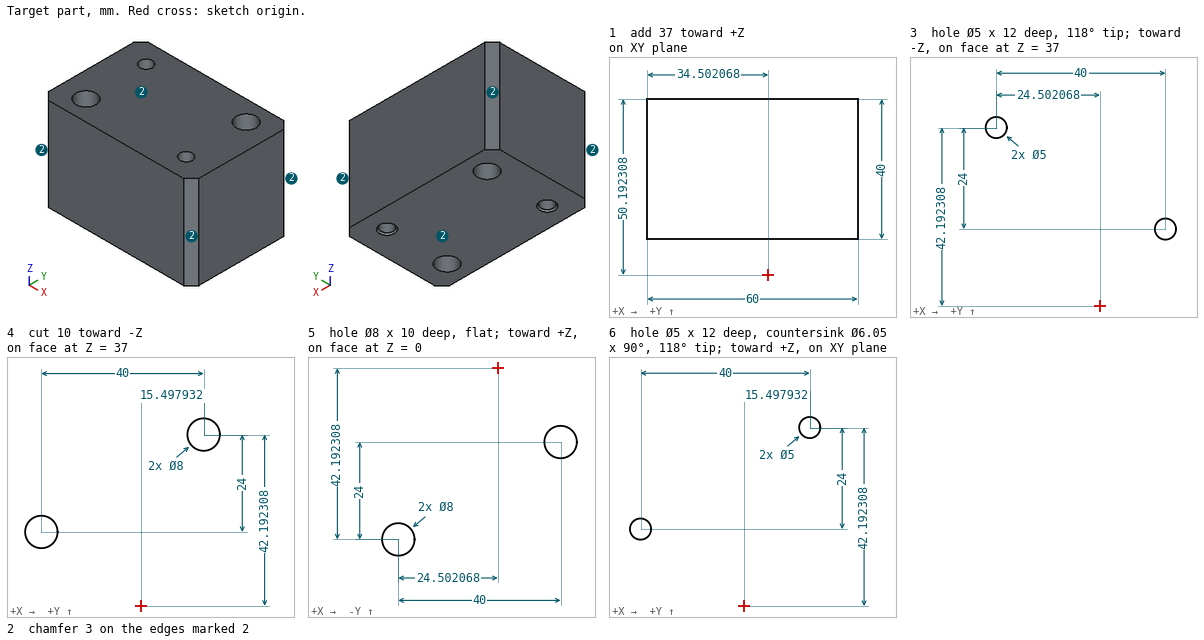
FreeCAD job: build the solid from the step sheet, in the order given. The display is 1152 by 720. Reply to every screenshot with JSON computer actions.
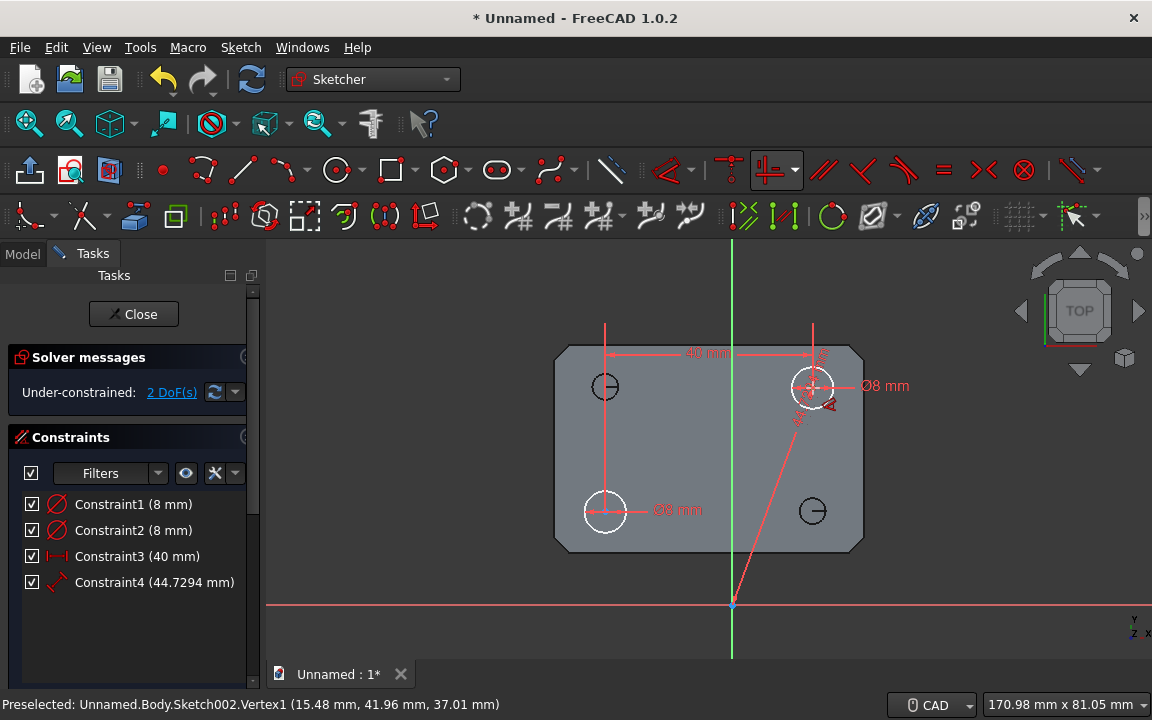
{"action": "left_click", "coordinate": [605, 512]}
{"action": "left_click", "coordinate": [571, 450]}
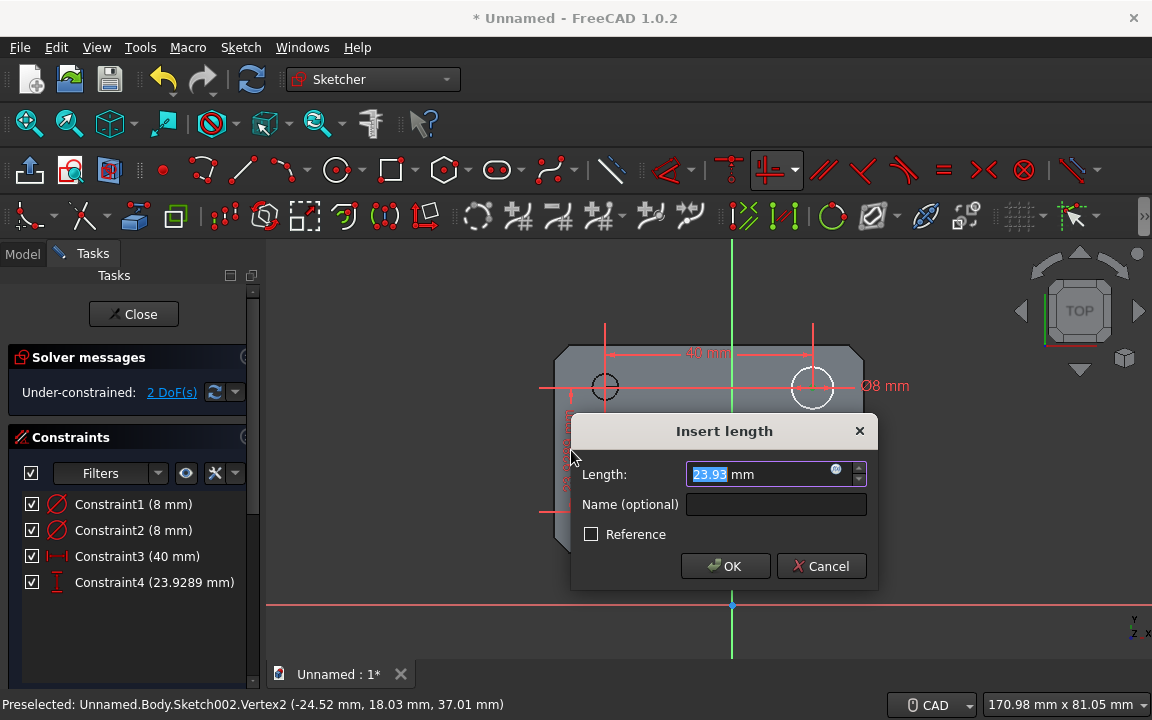
{"action": "type", "text": "24"}
{"action": "key", "text": "Return"}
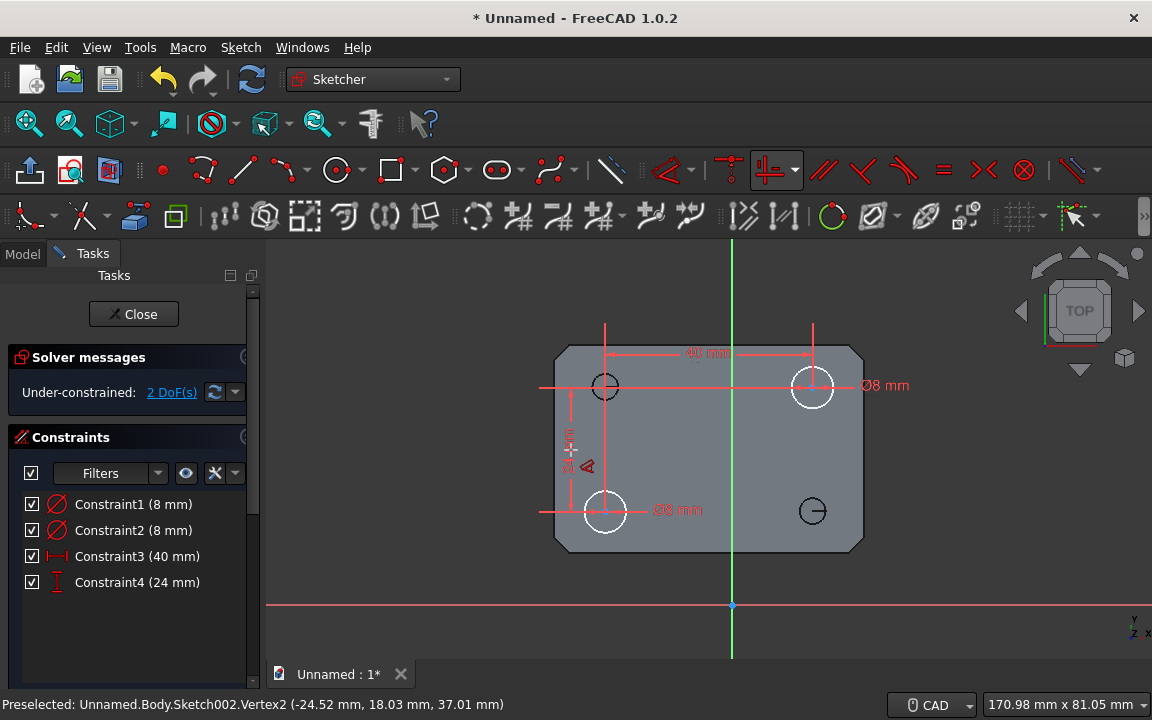
{"action": "left_click", "coordinate": [813, 388]}
{"action": "left_click", "coordinate": [791, 354]}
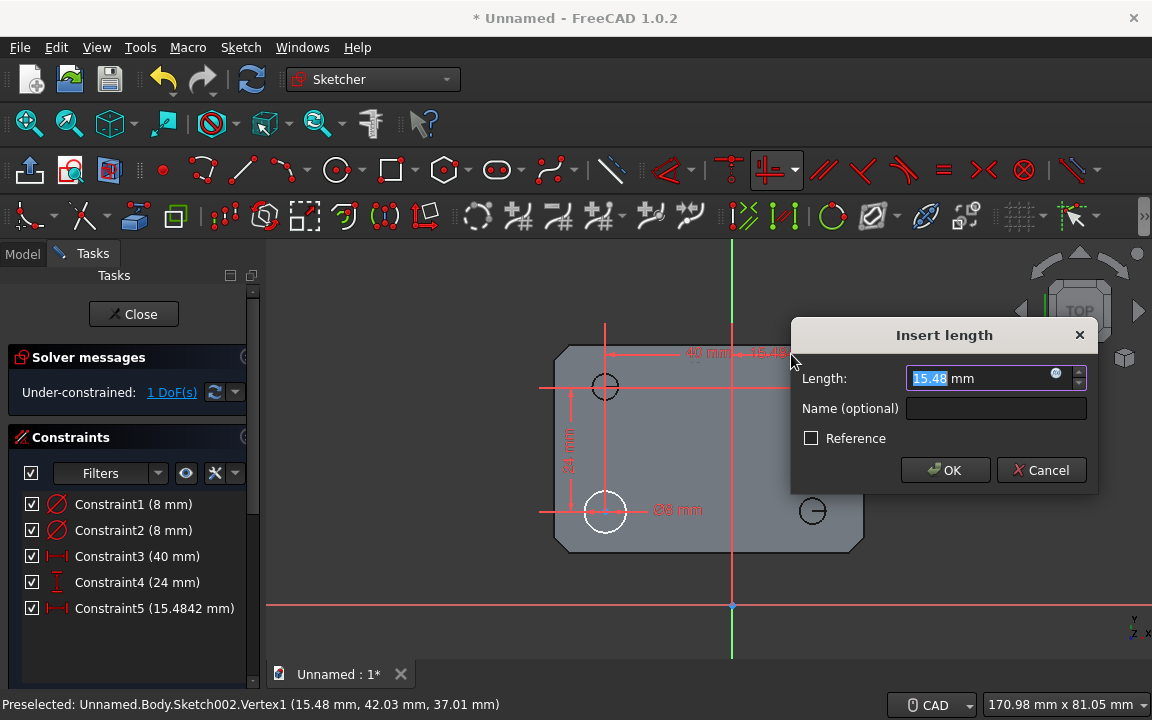
{"action": "type", "text": "15.497932"}
{"action": "key", "text": "Return"}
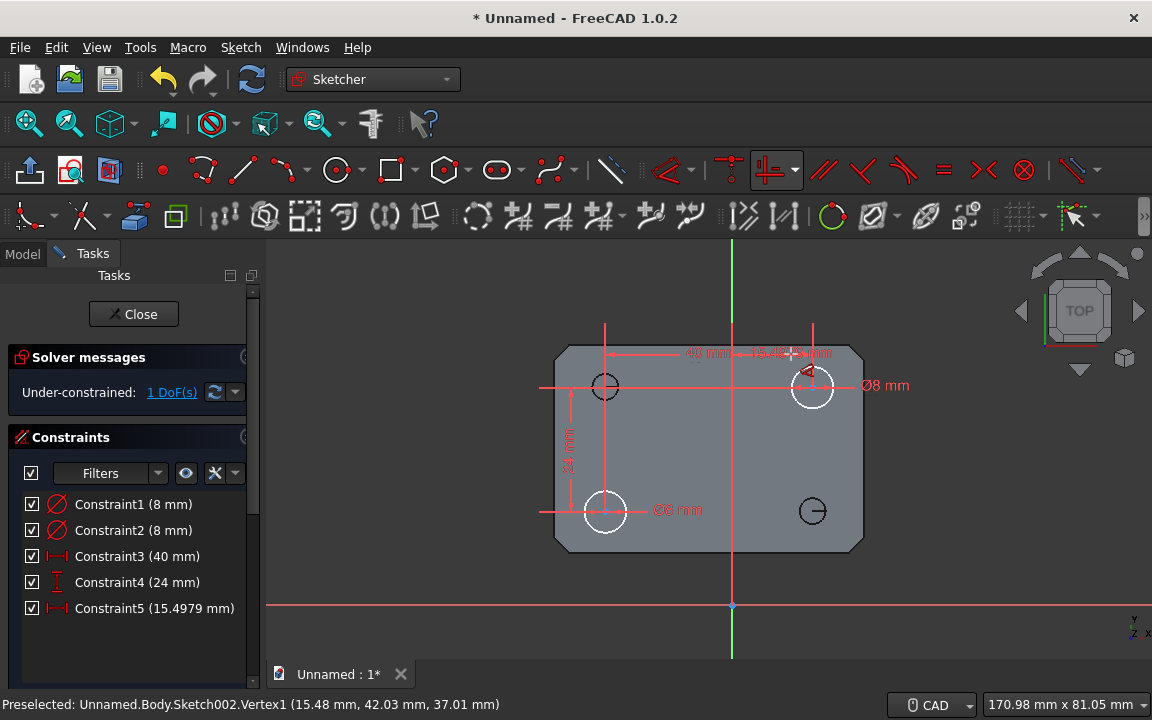
{"action": "left_click", "coordinate": [813, 388]}
{"action": "left_click", "coordinate": [847, 497]}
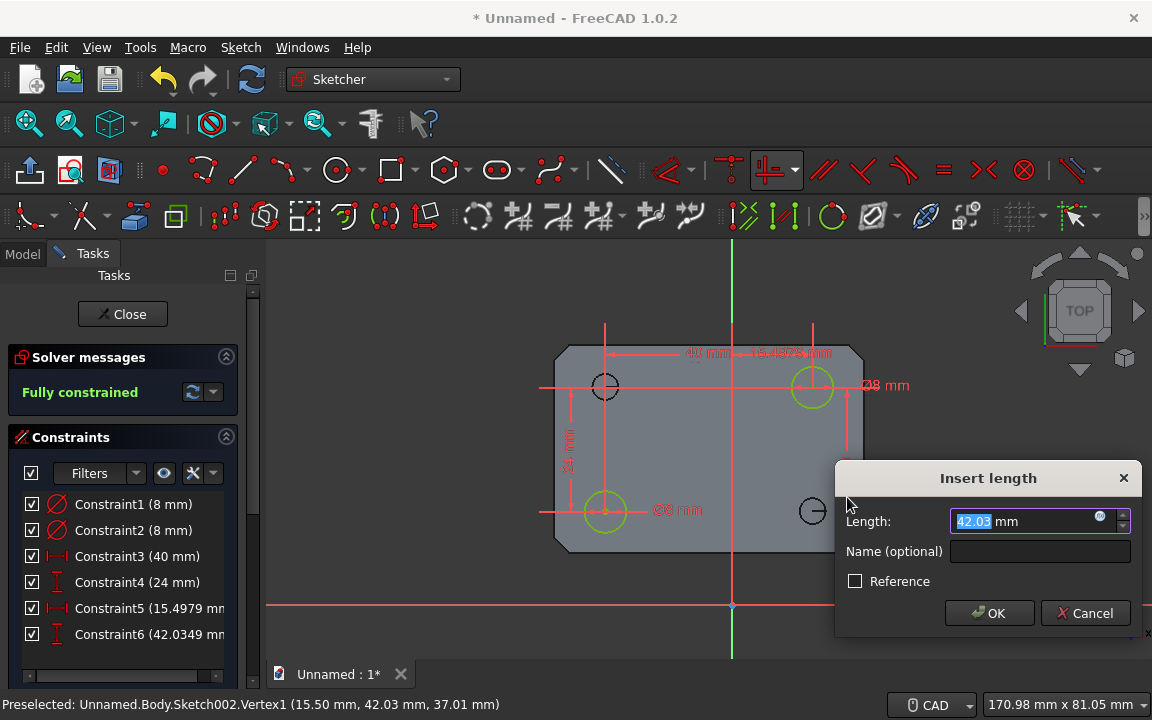
{"action": "type", "text": "42.192308"}
{"action": "key", "text": "Return"}
{"action": "key", "text": "Escape"}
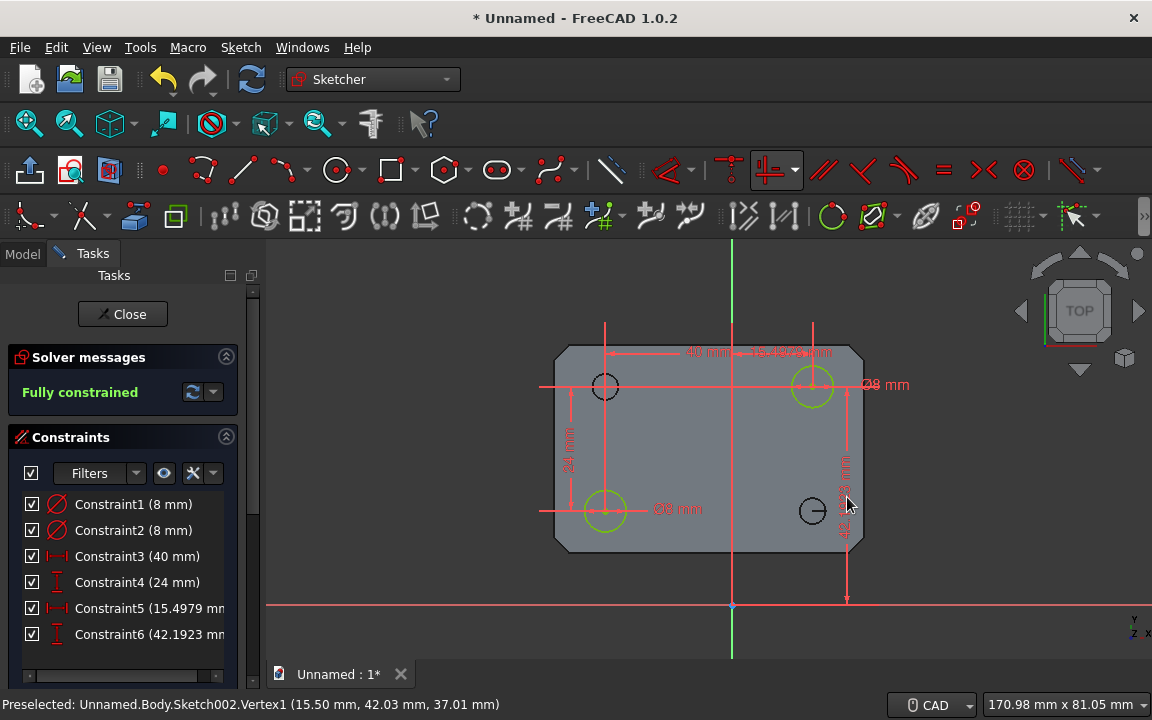
{"action": "left_click", "coordinate": [123, 314]}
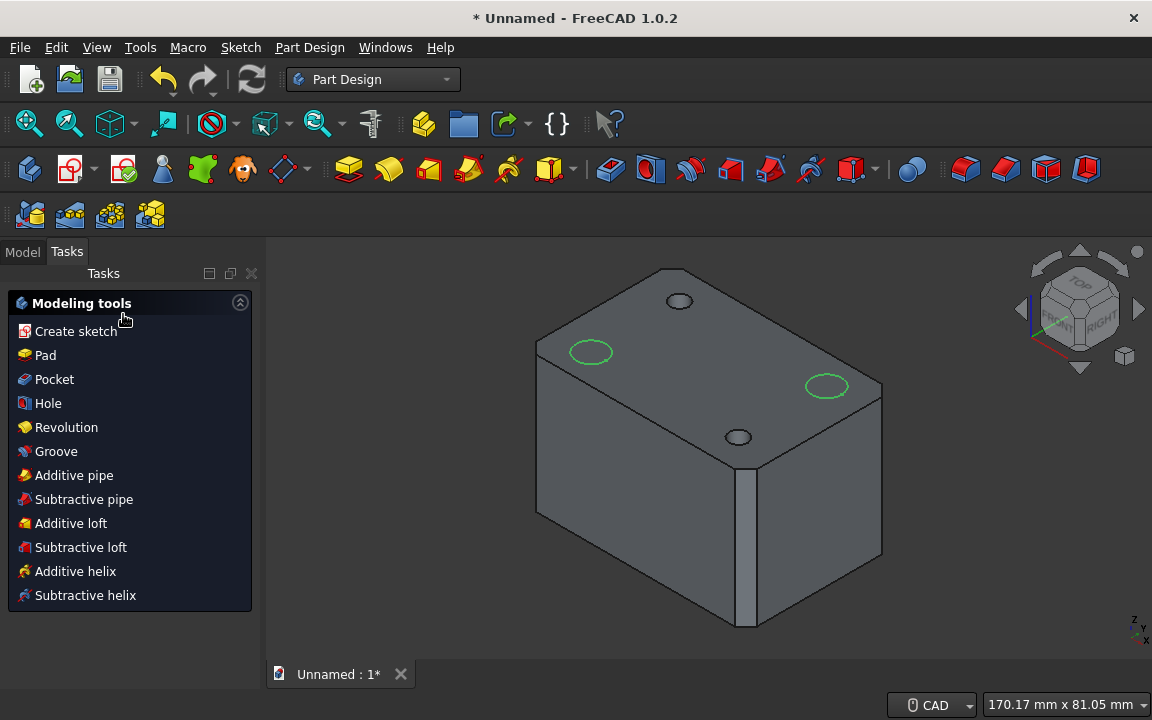
{"action": "left_click", "coordinate": [612, 170]}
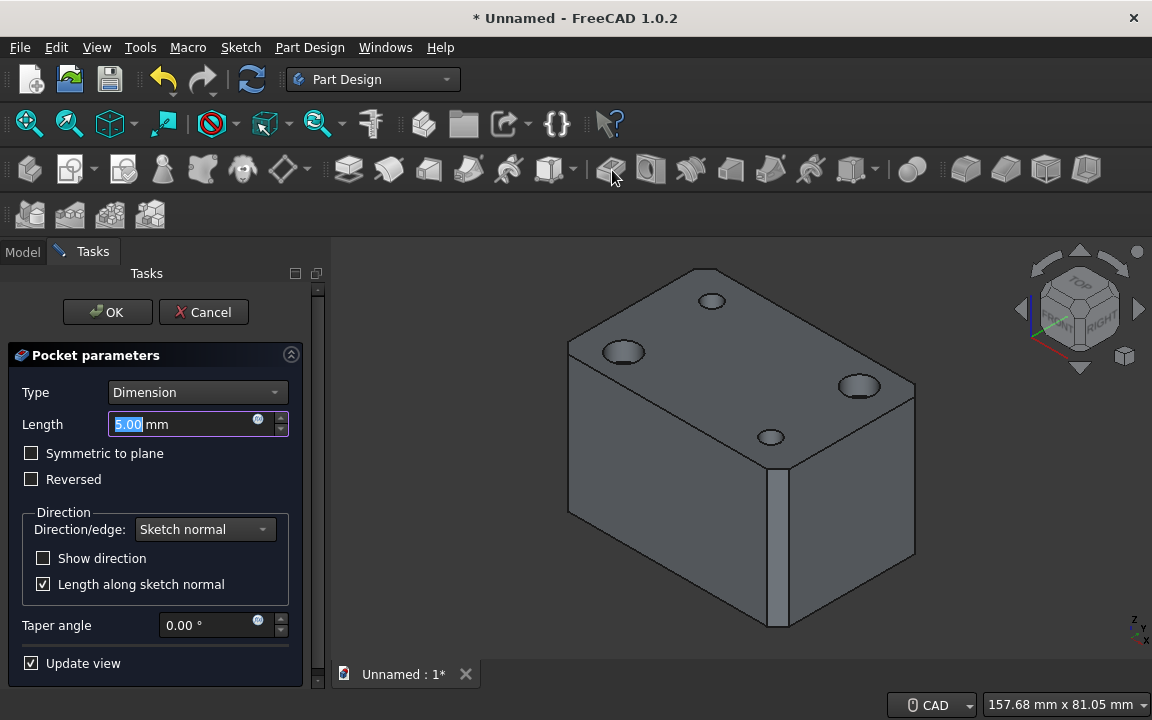
{"action": "type", "text": "10"}
{"action": "key", "text": "Tab"}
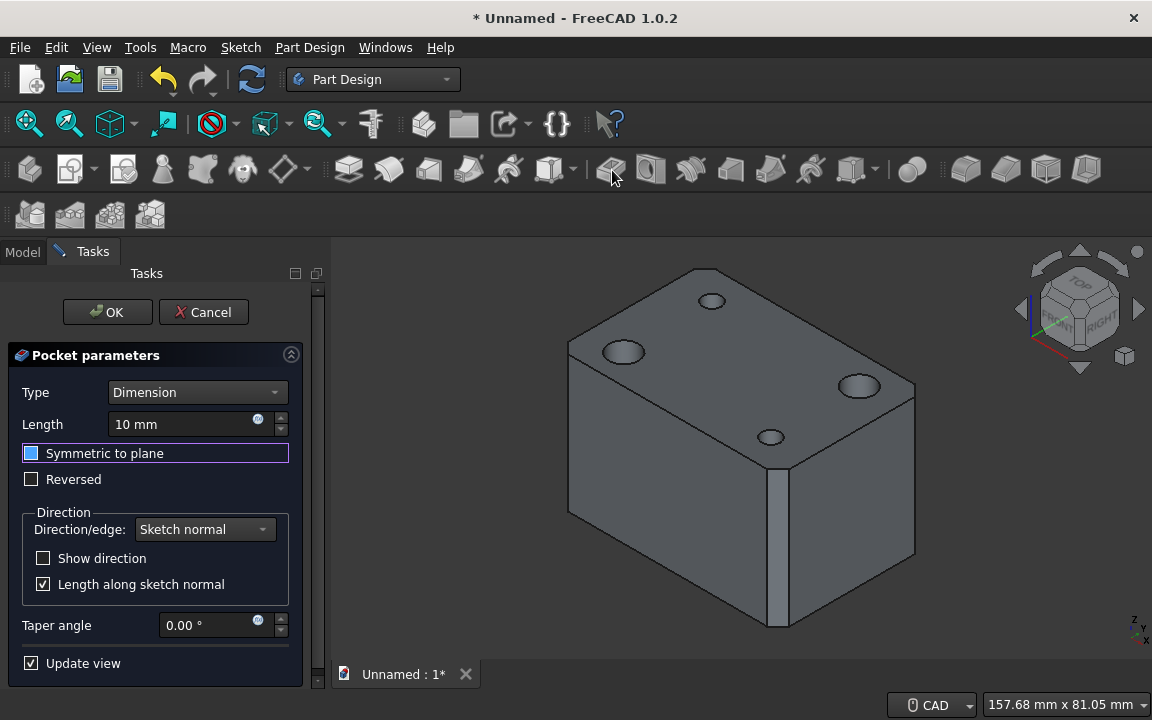
{"action": "left_click", "coordinate": [108, 312]}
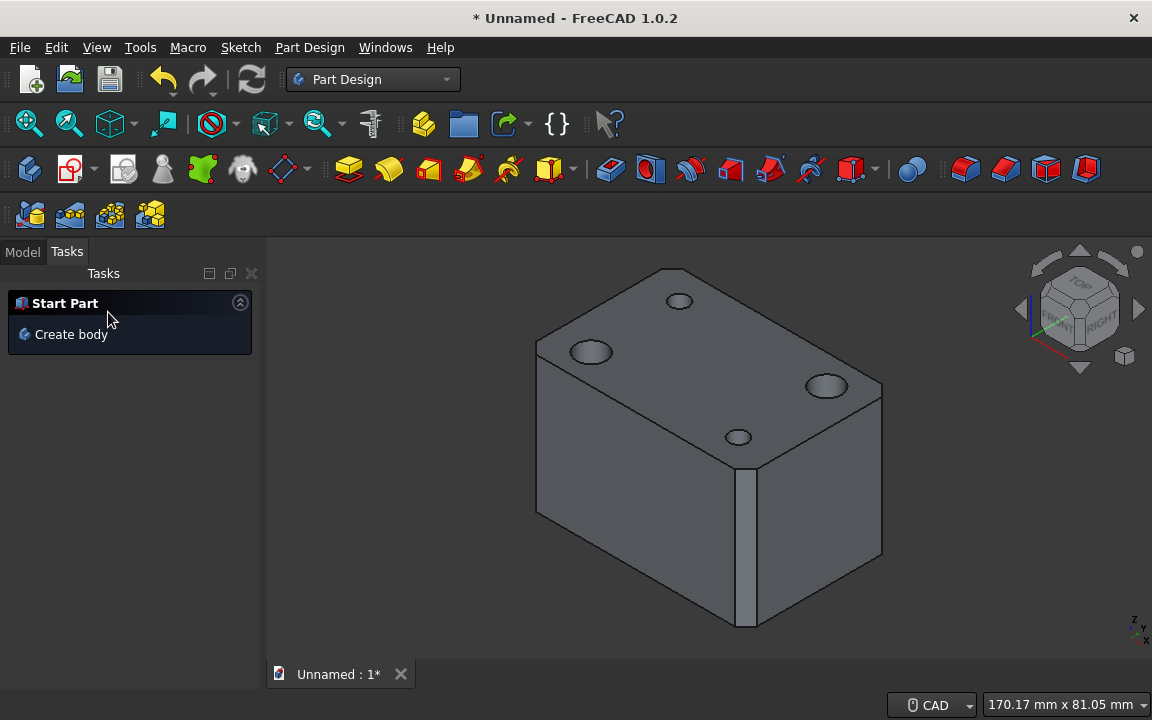
{"action": "key", "text": "5"}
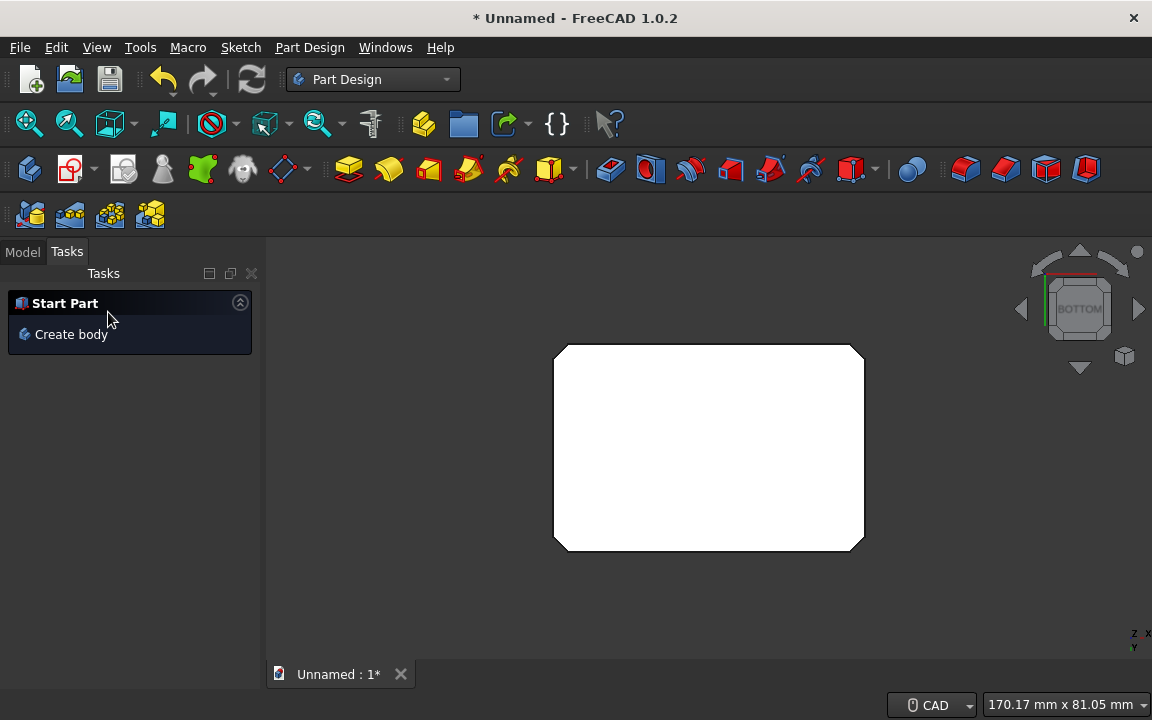
{"action": "left_click", "coordinate": [754, 447]}